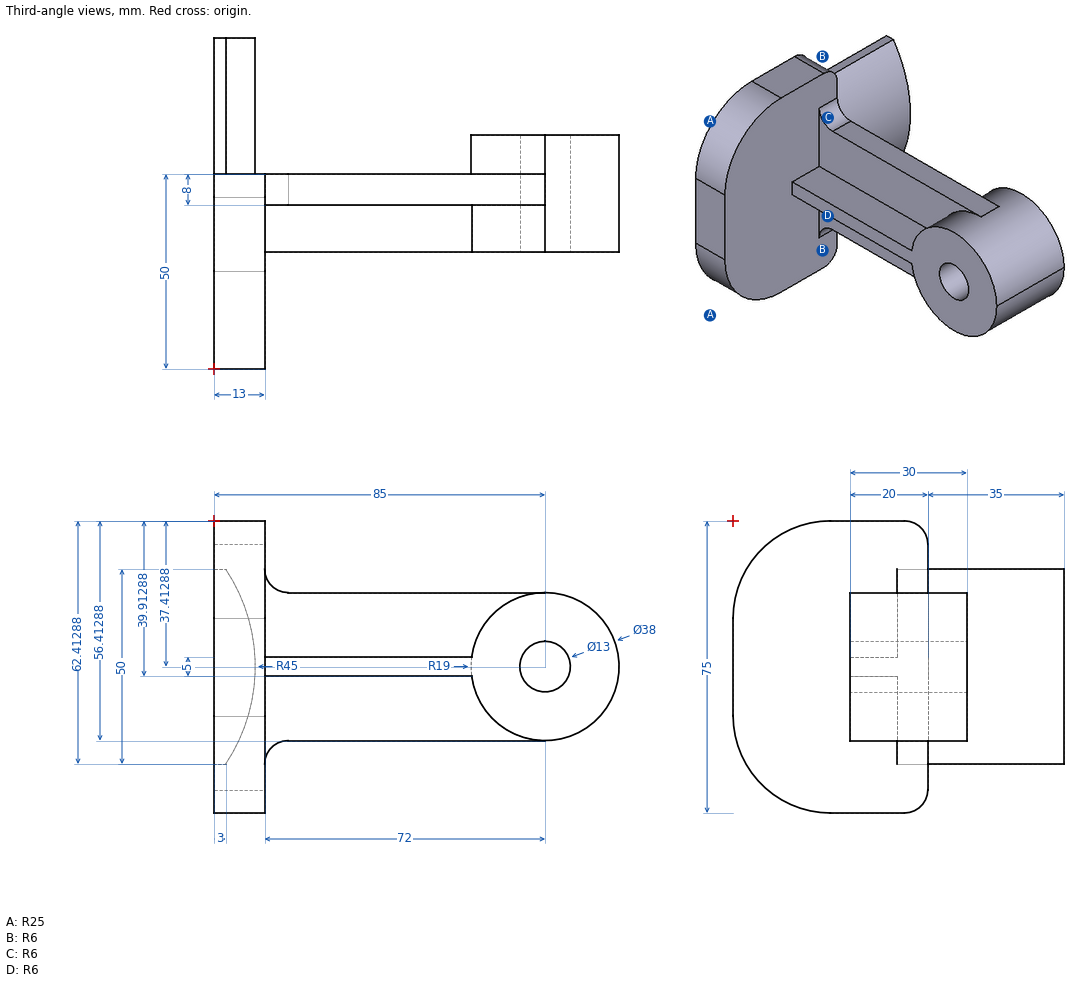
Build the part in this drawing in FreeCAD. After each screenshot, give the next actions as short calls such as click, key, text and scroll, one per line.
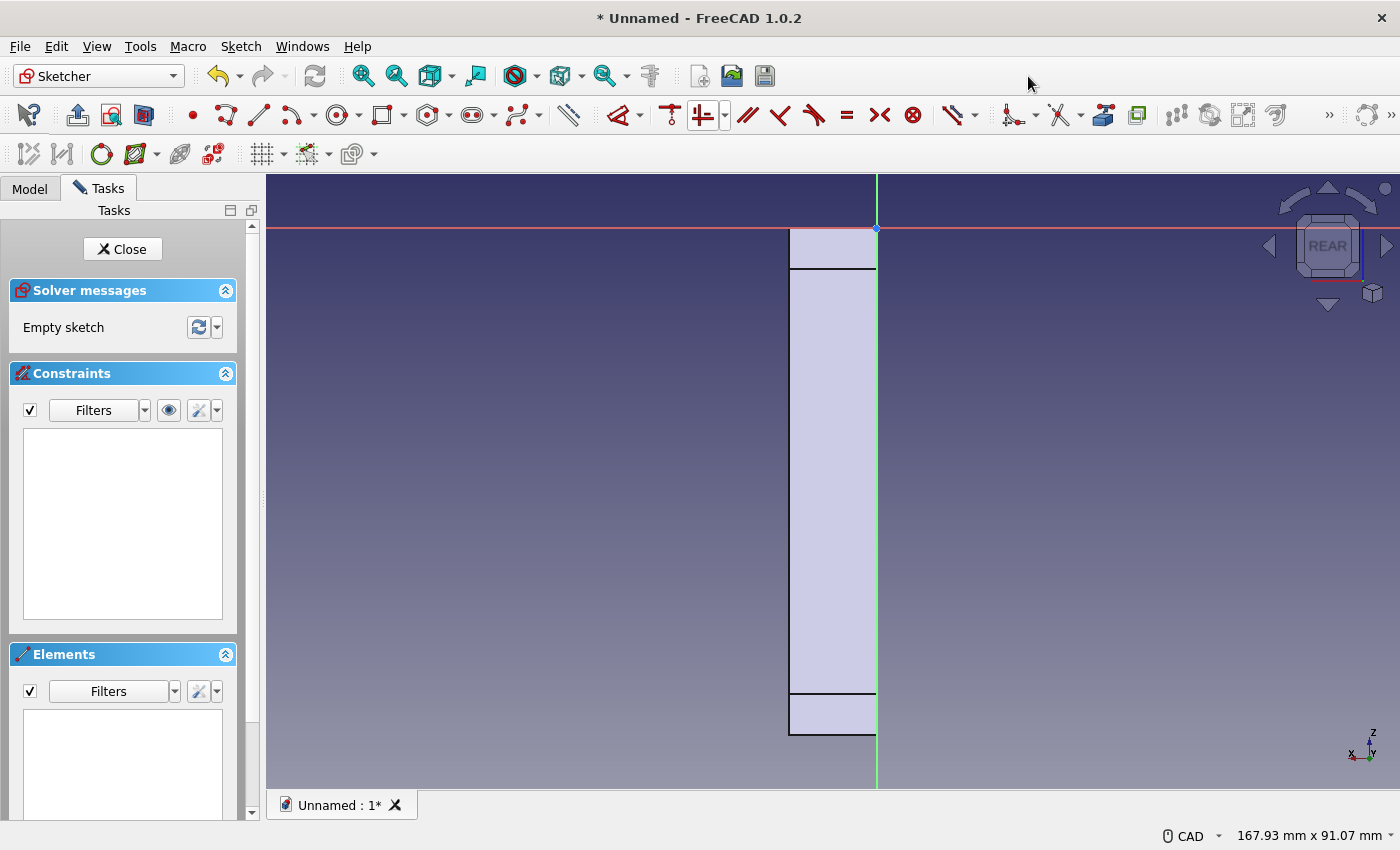
click(226, 116)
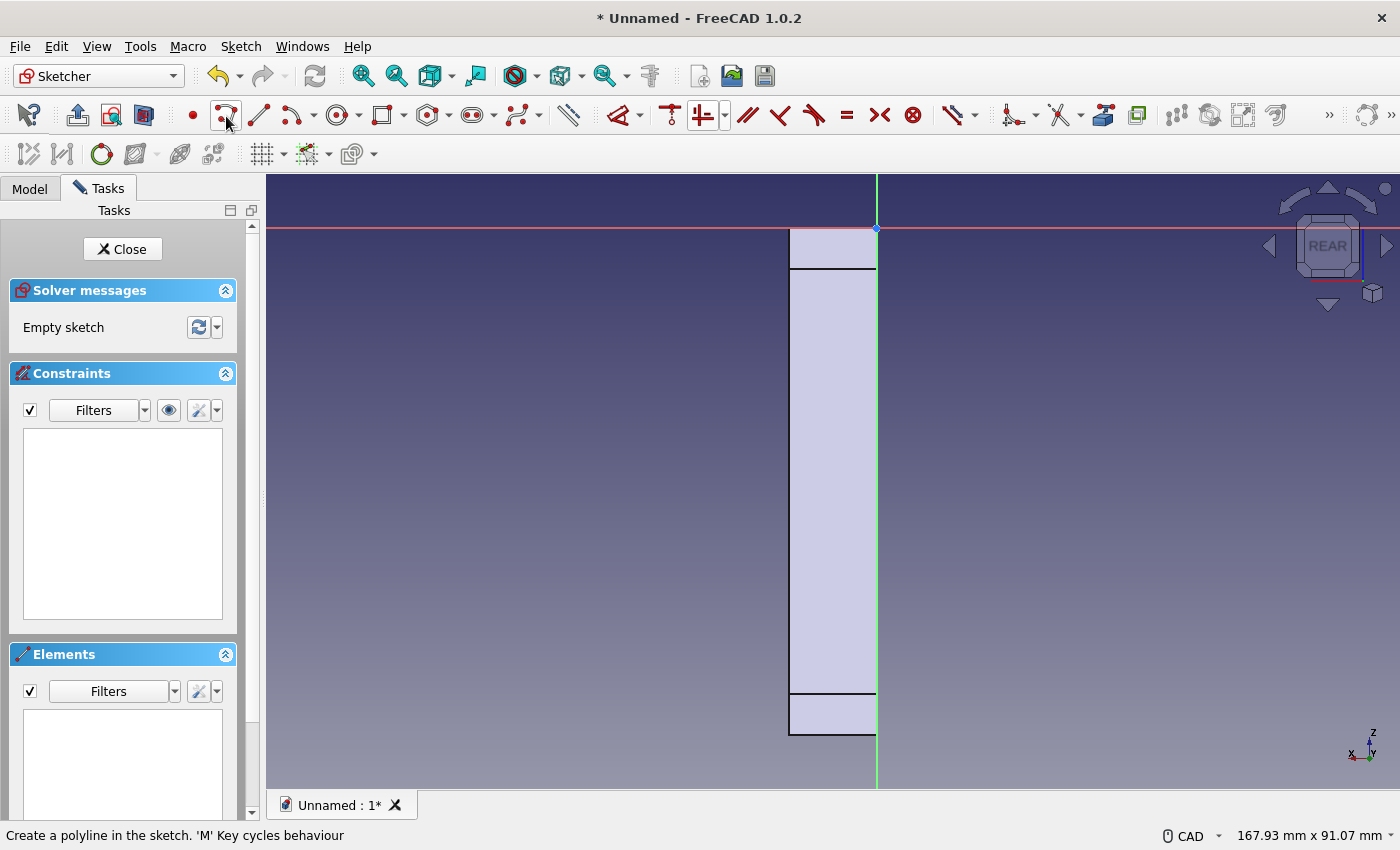
click(857, 650)
click(877, 650)
click(868, 312)
click(857, 312)
right_click(857, 312)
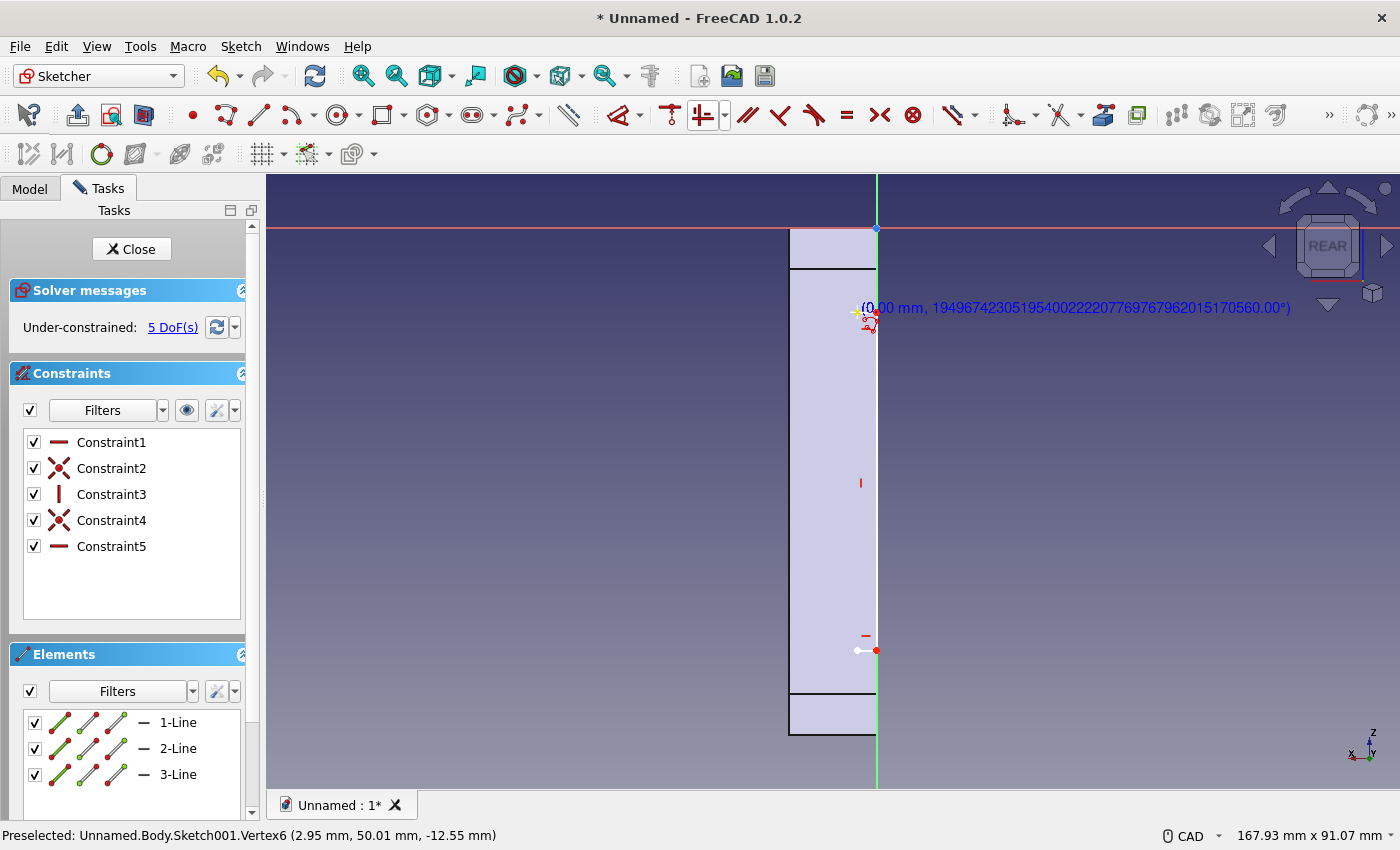
click(314, 116)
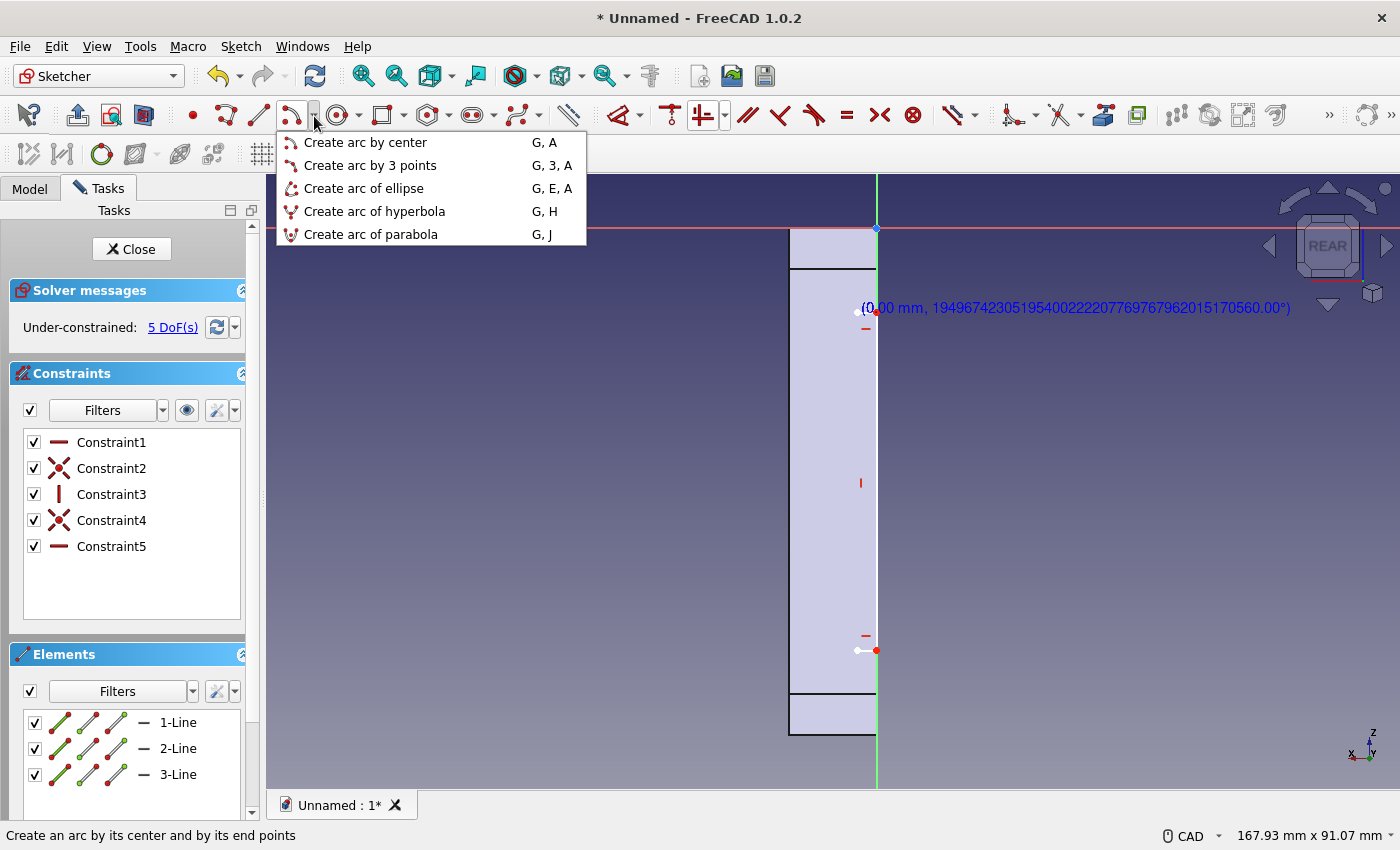
click(432, 166)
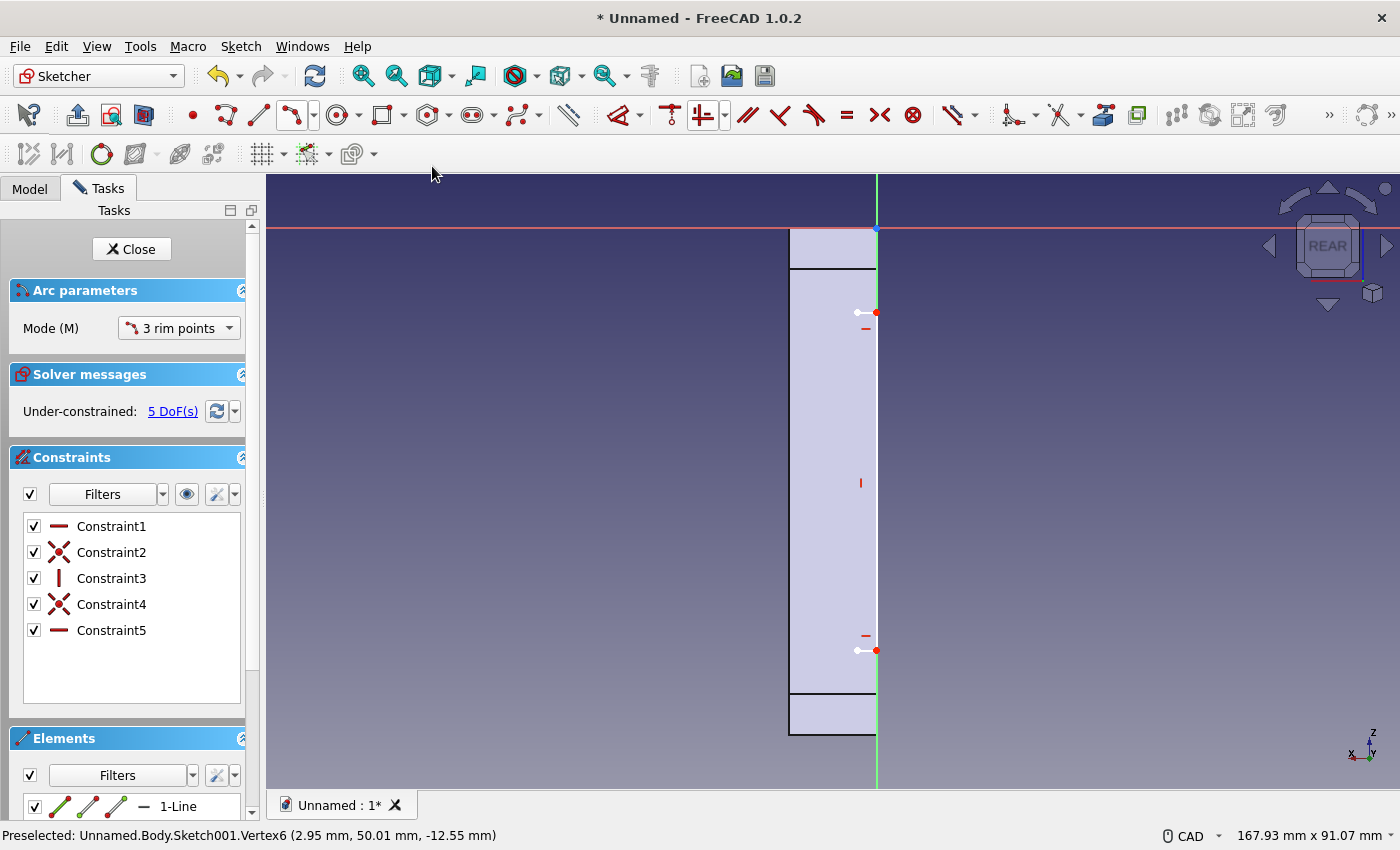
scroll(857, 312, up, 3)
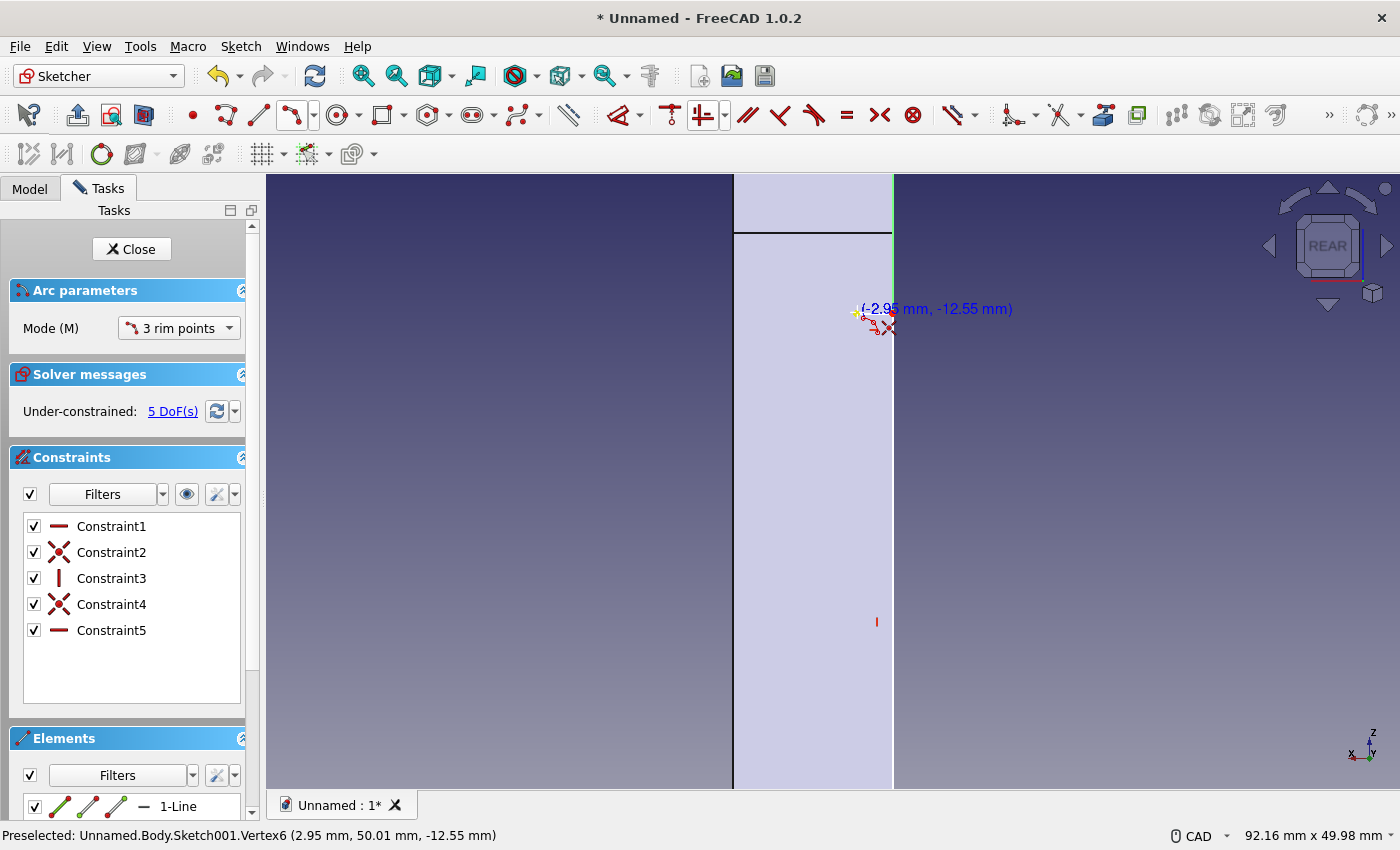
click(857, 314)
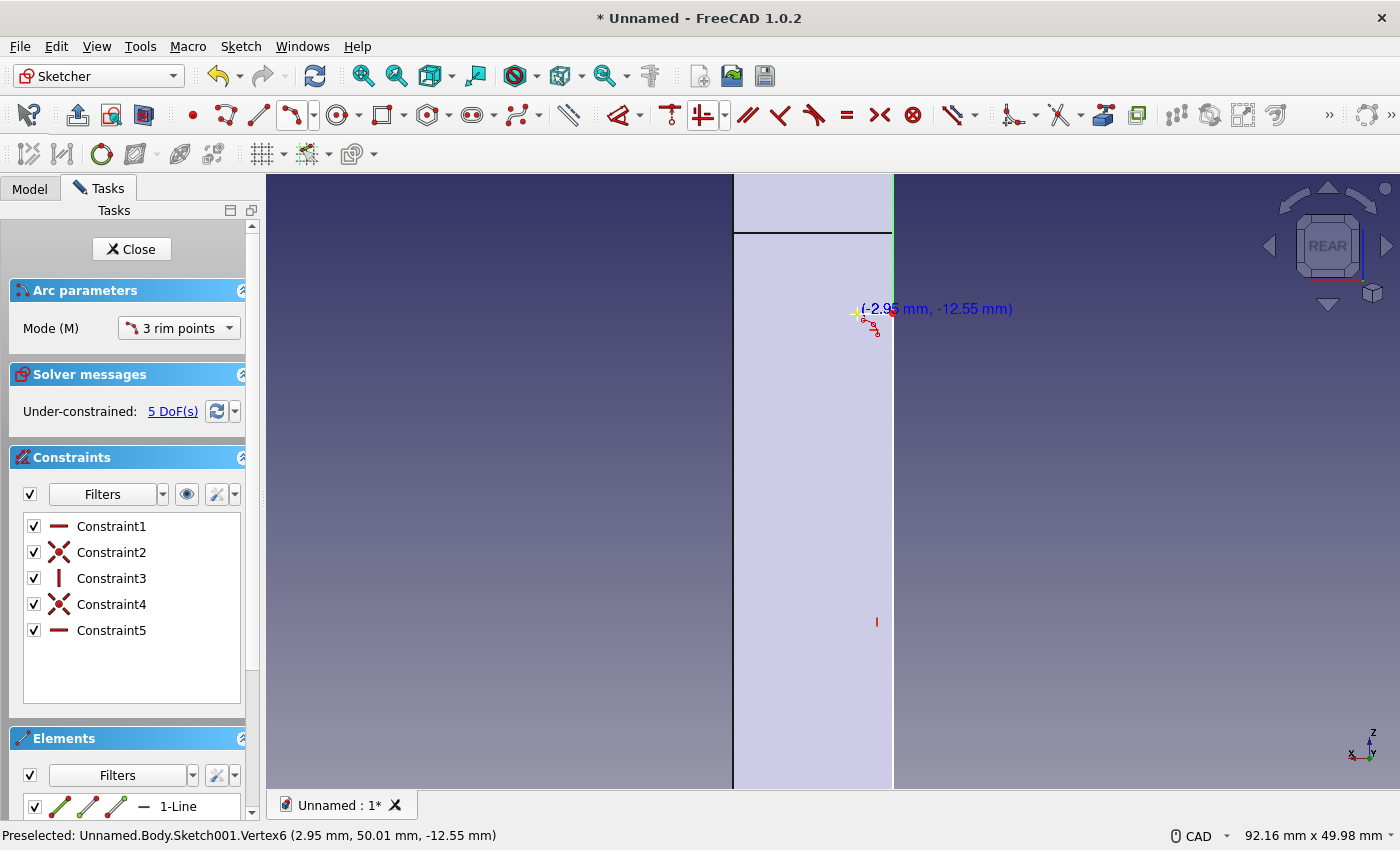
scroll(688, 406, down, 3)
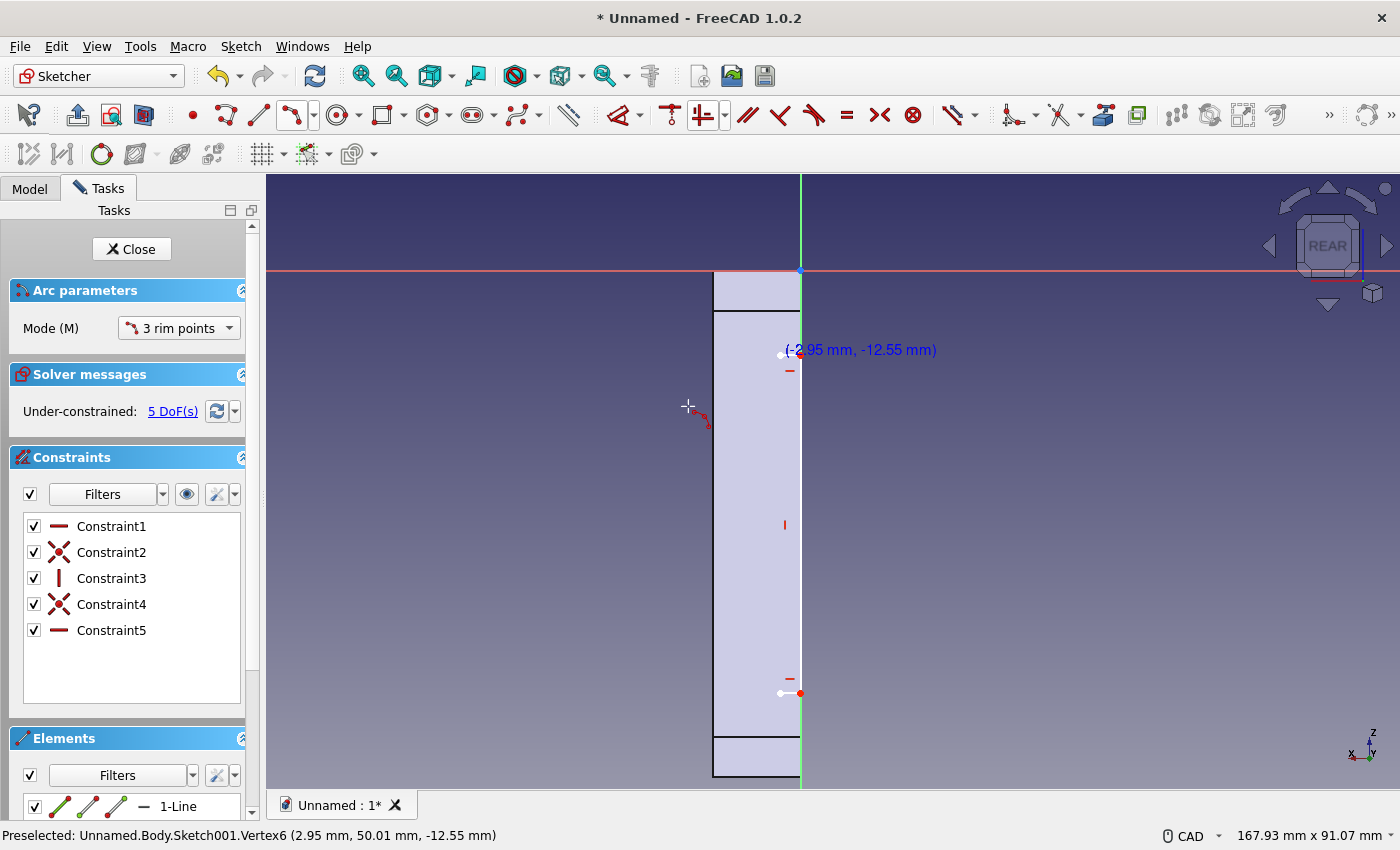
scroll(780, 692, up, 3)